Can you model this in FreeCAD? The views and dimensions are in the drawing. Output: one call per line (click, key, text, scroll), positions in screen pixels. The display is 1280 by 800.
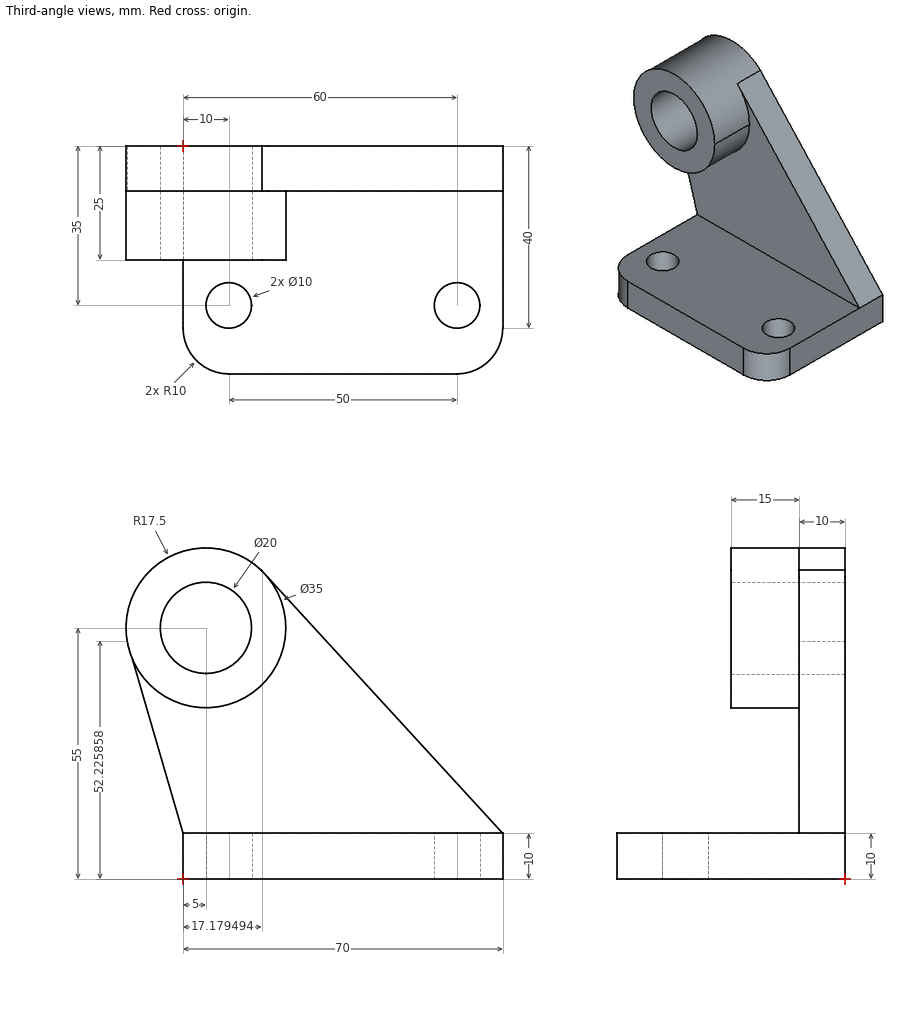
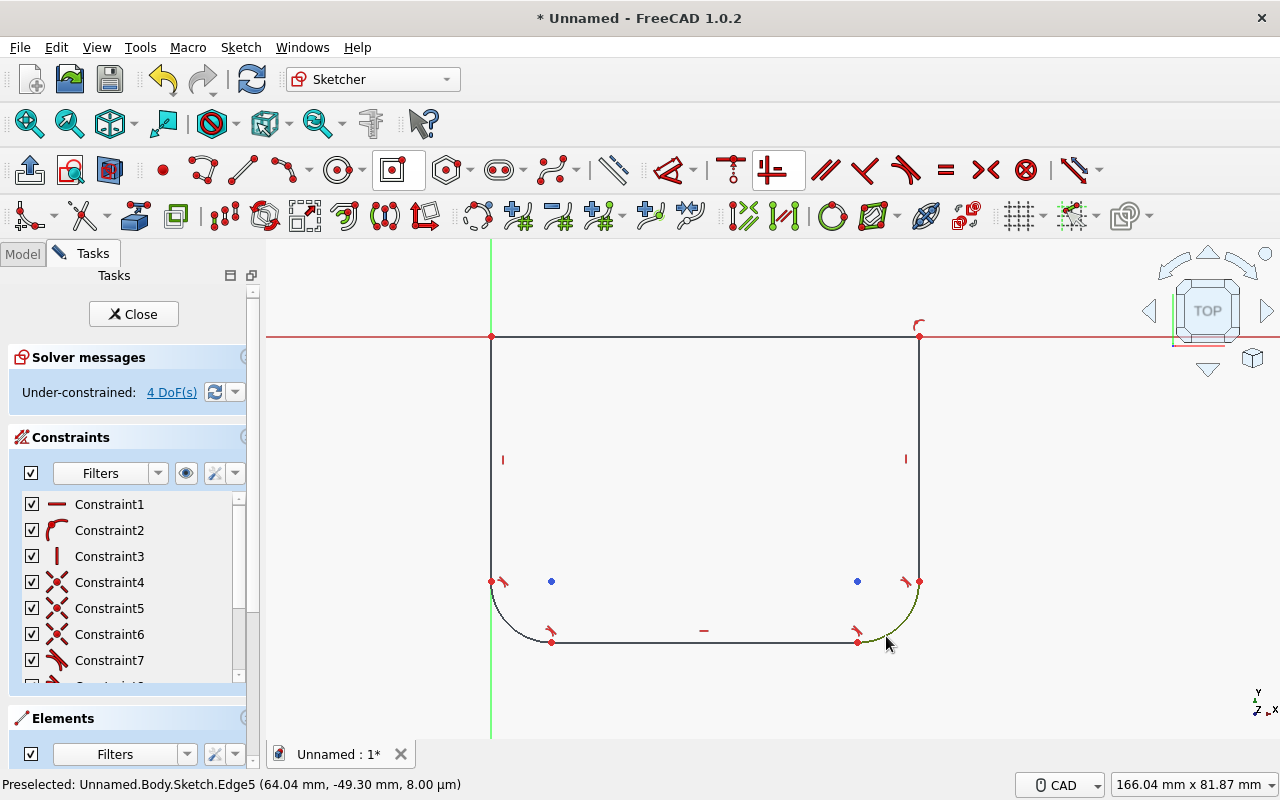
click(524, 636)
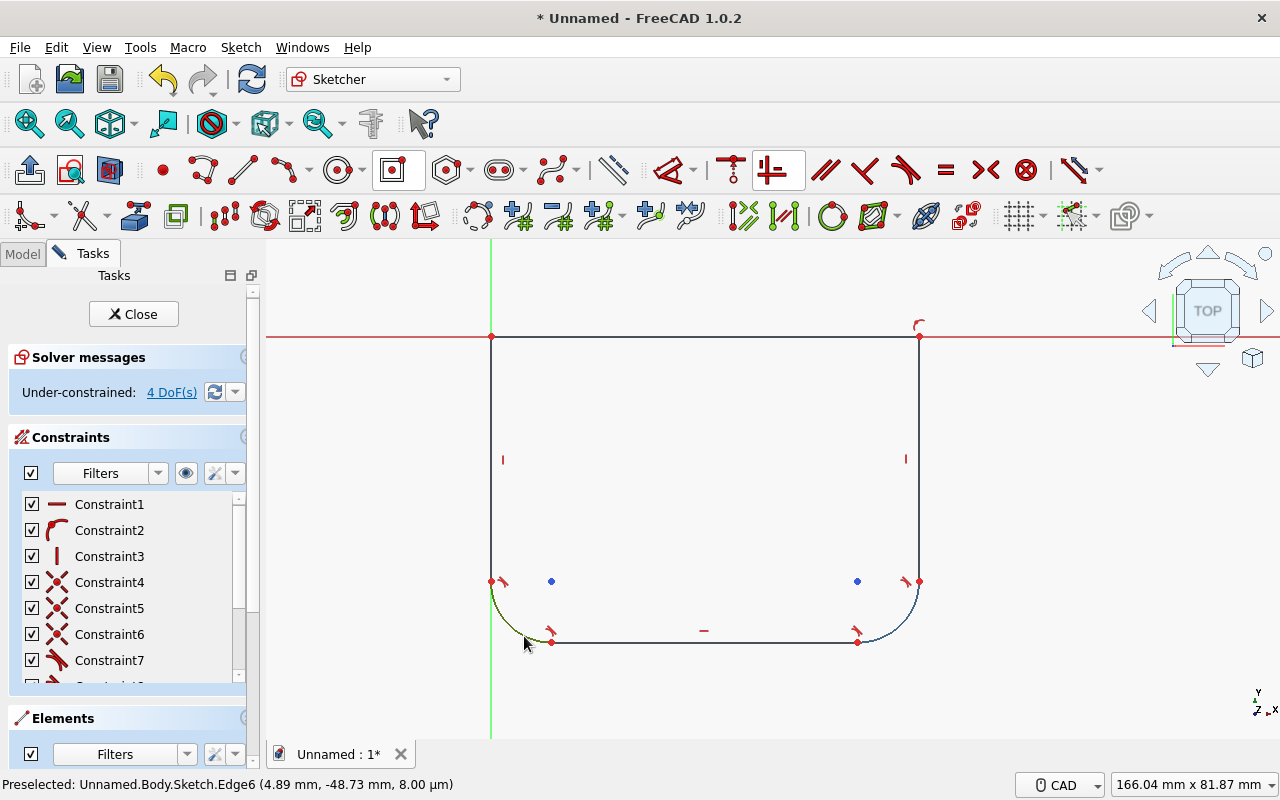
click(946, 170)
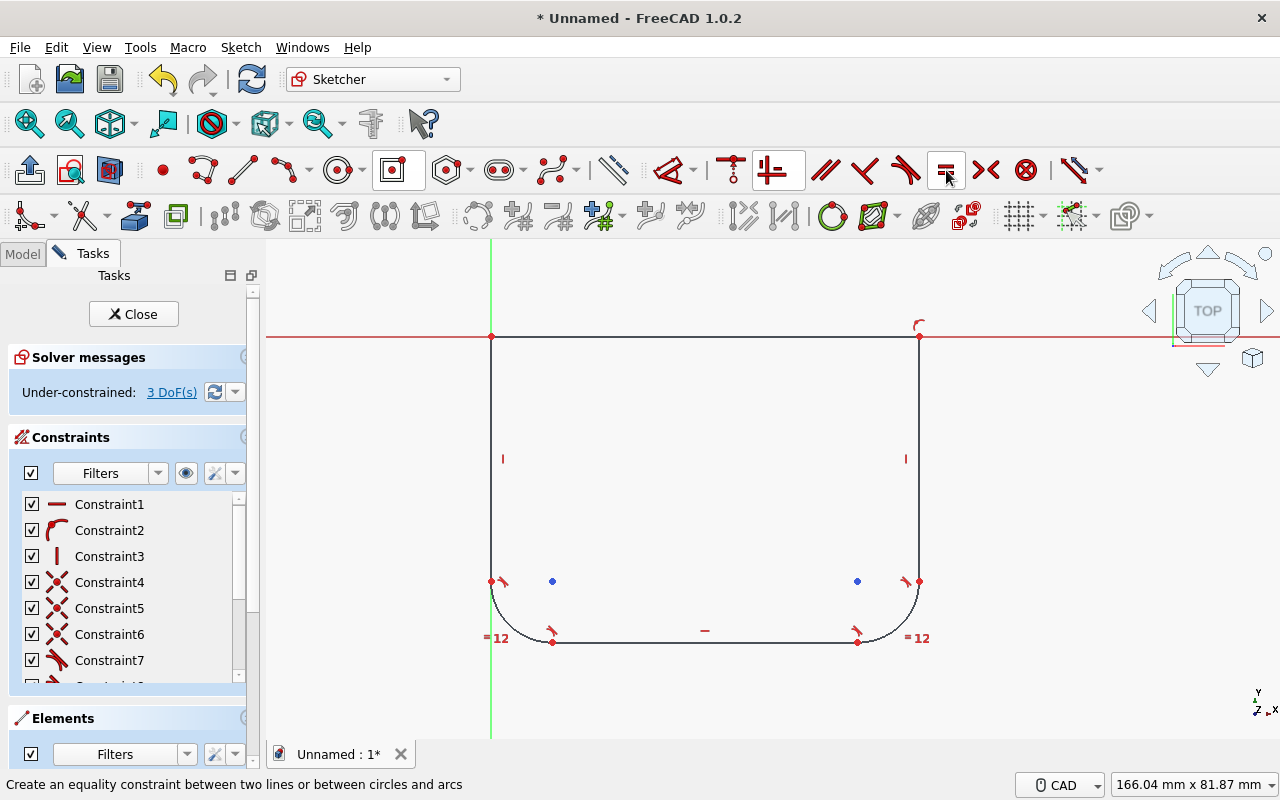
click(668, 170)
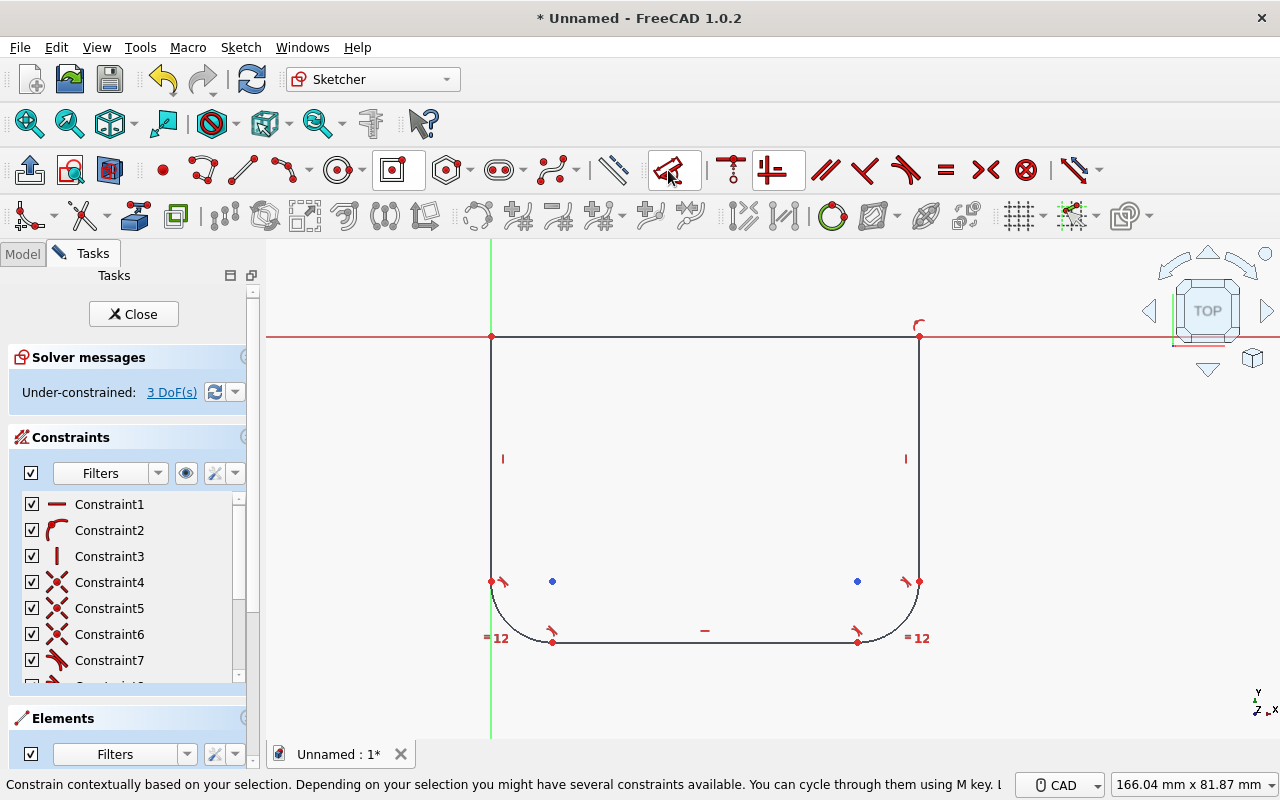
click(886, 636)
click(901, 664)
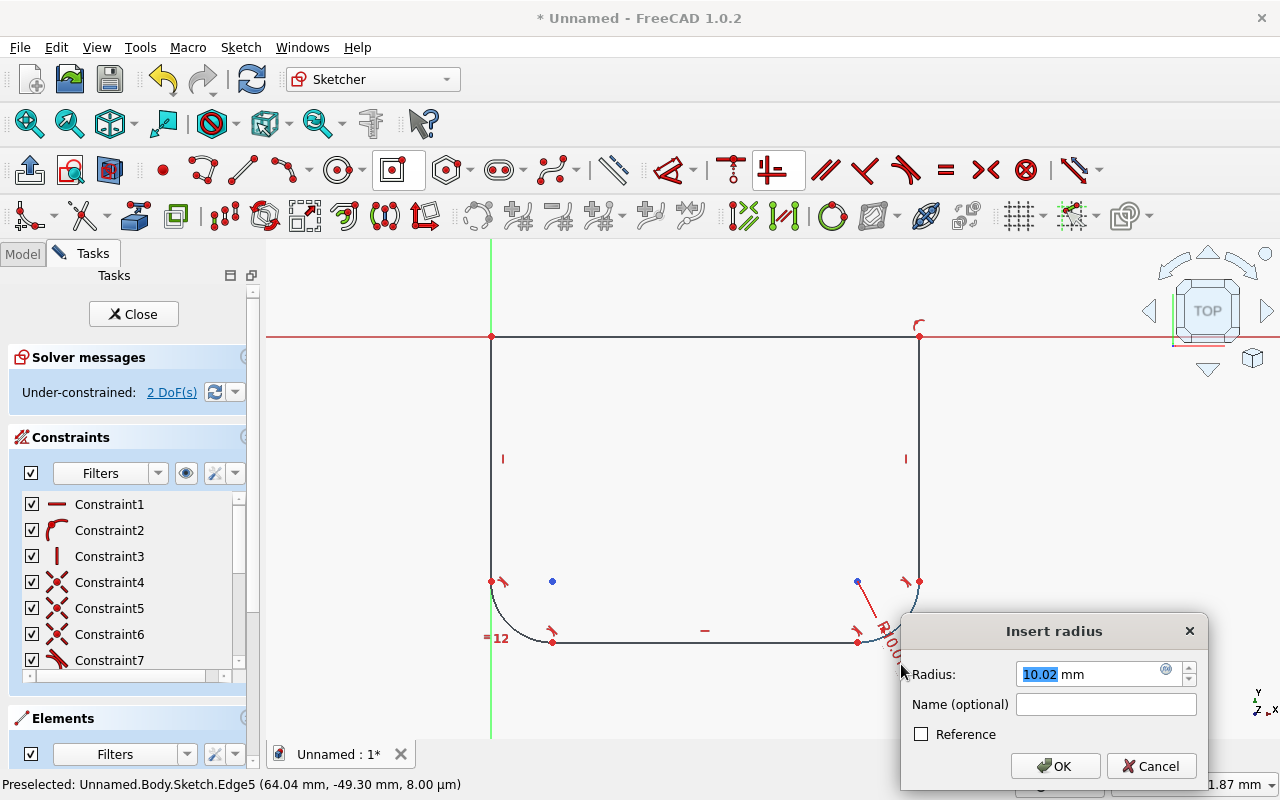
text(10)
key(Return)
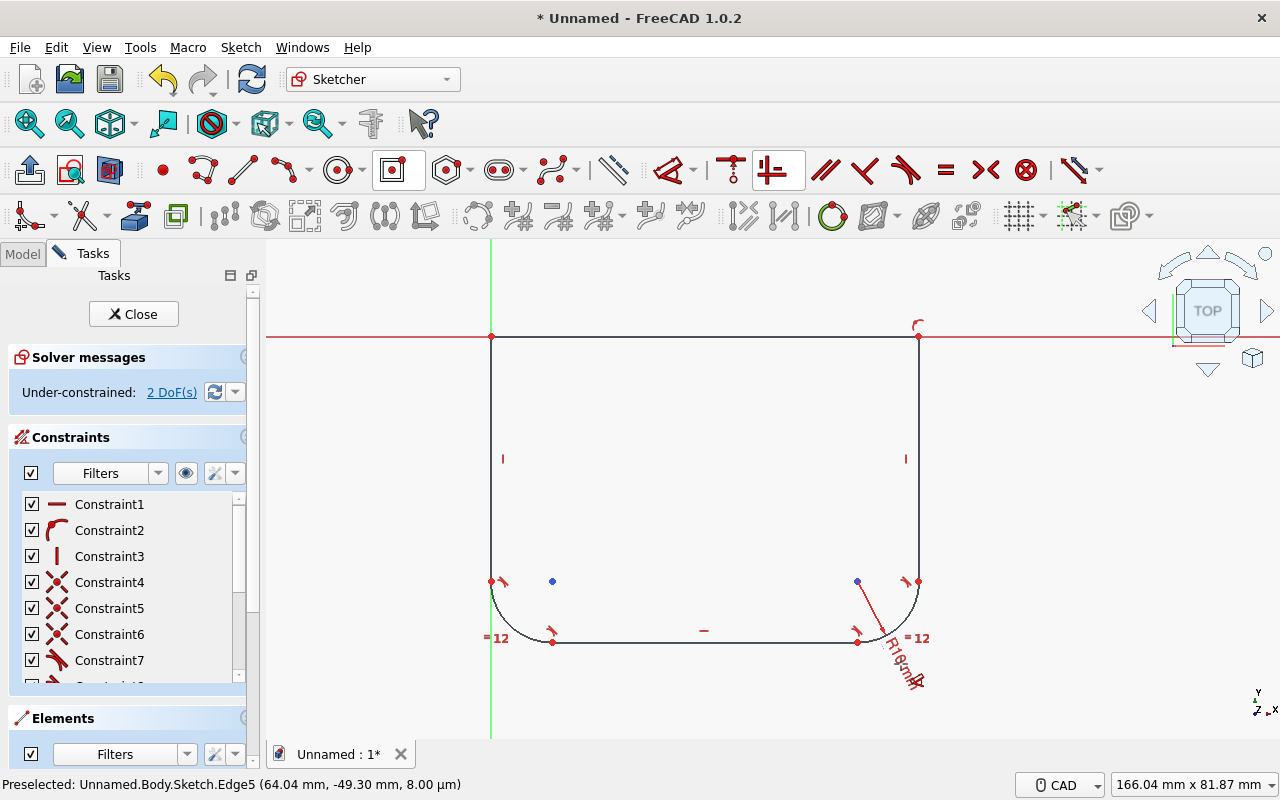
click(644, 643)
click(705, 677)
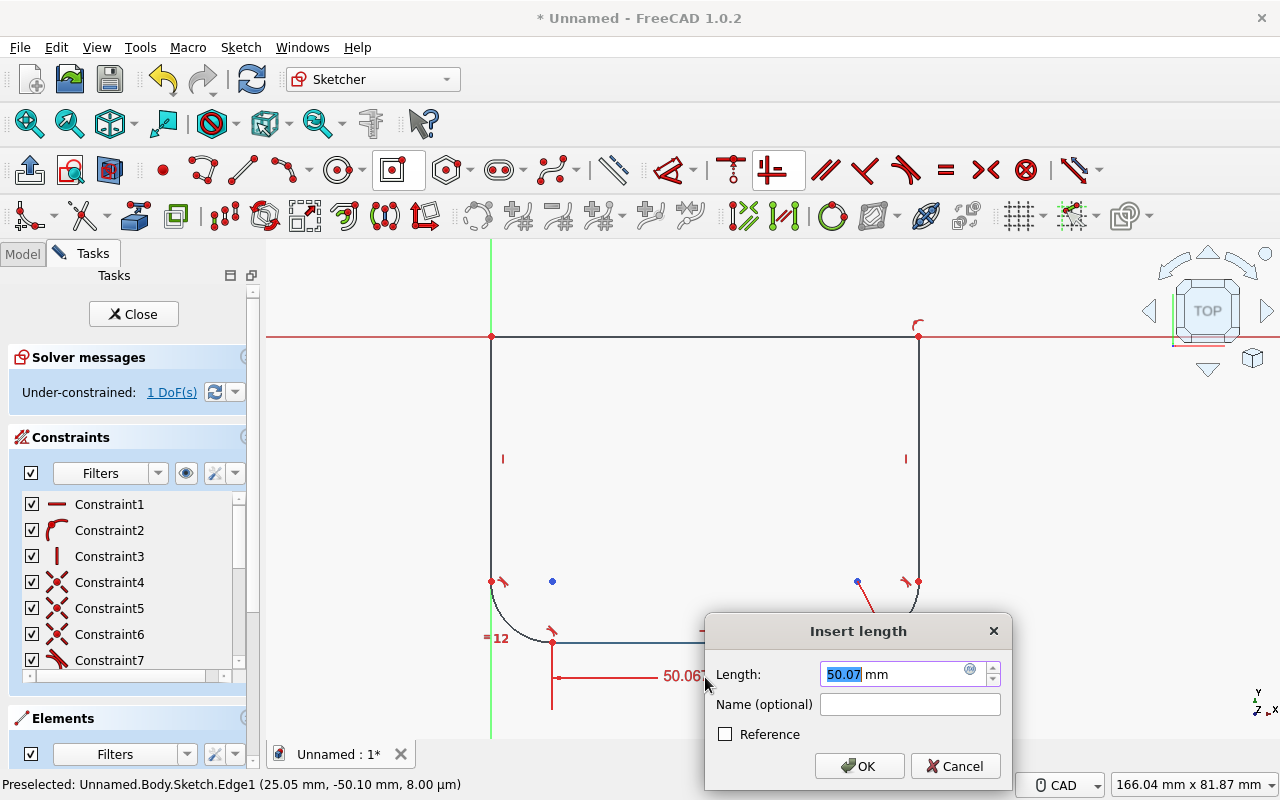
text(50)
key(Return)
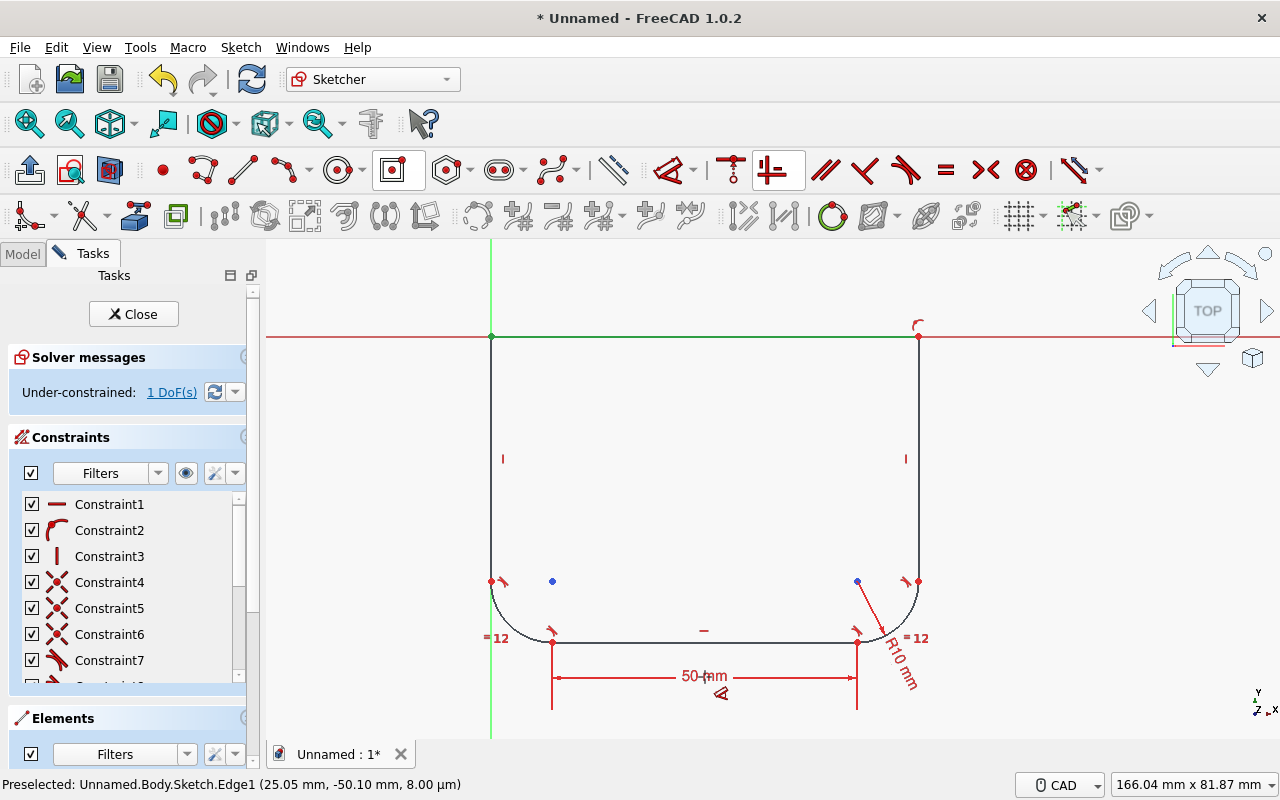
click(919, 508)
click(953, 459)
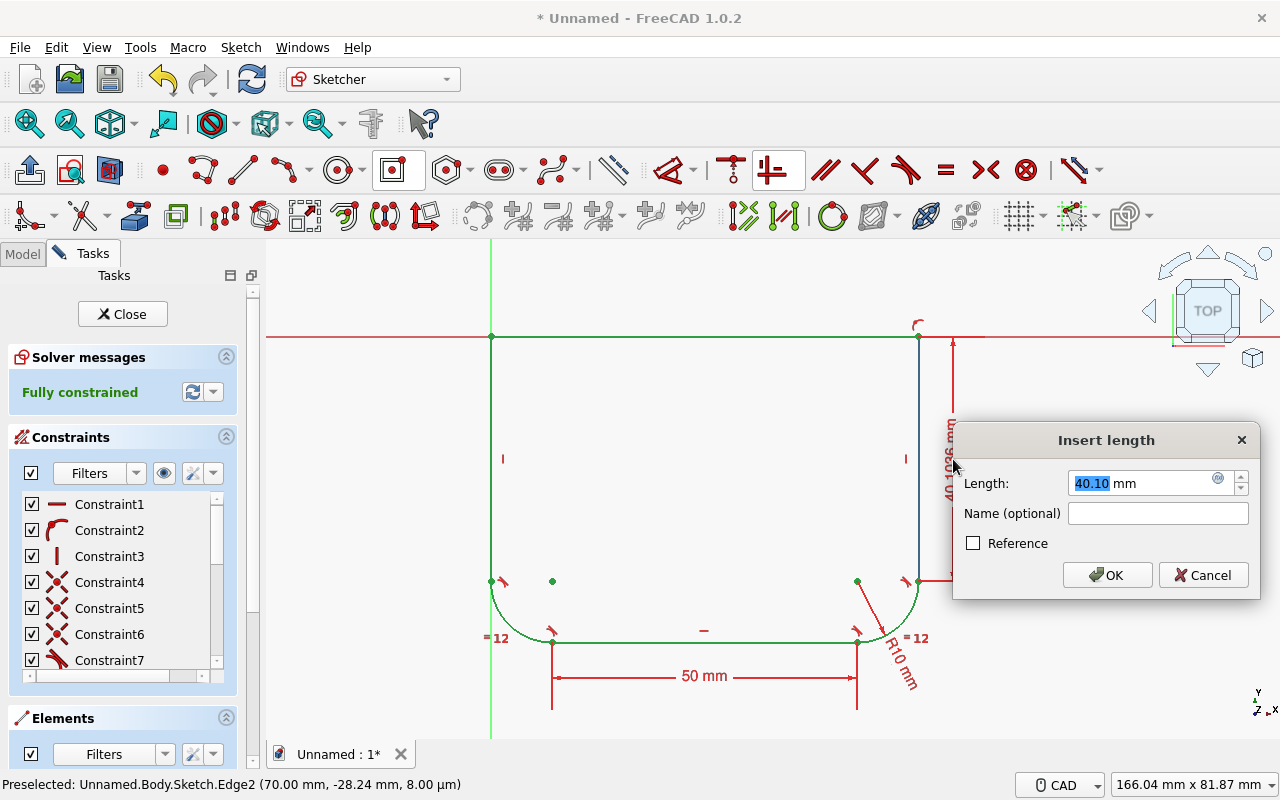
text(40)
key(Return)
key(Escape)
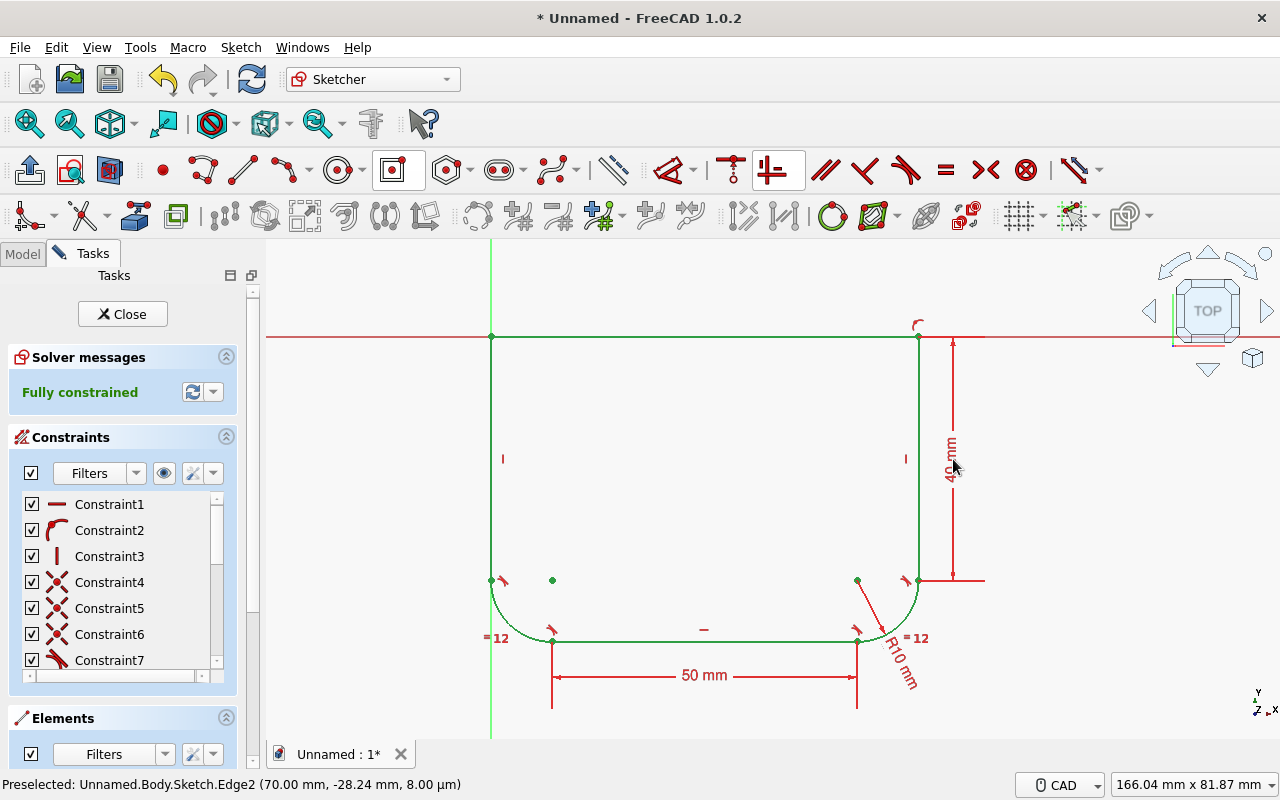
click(123, 314)